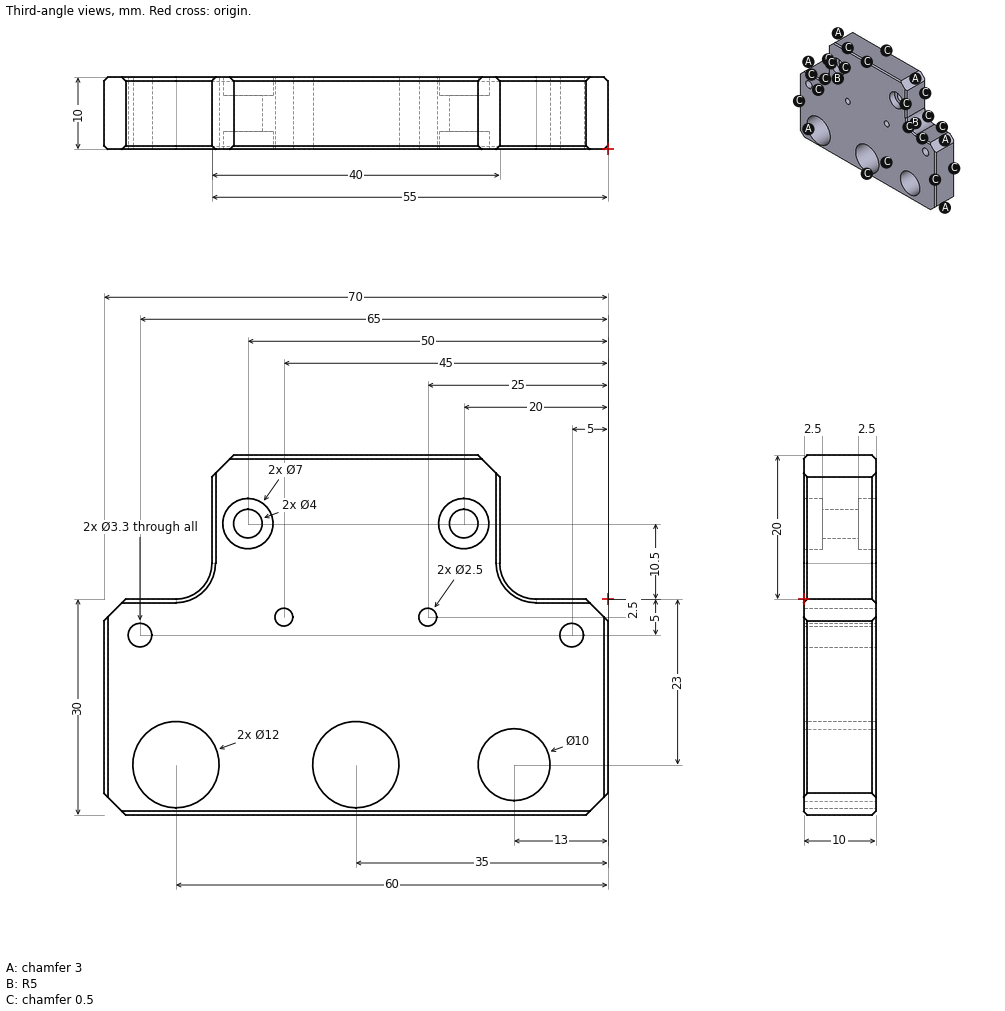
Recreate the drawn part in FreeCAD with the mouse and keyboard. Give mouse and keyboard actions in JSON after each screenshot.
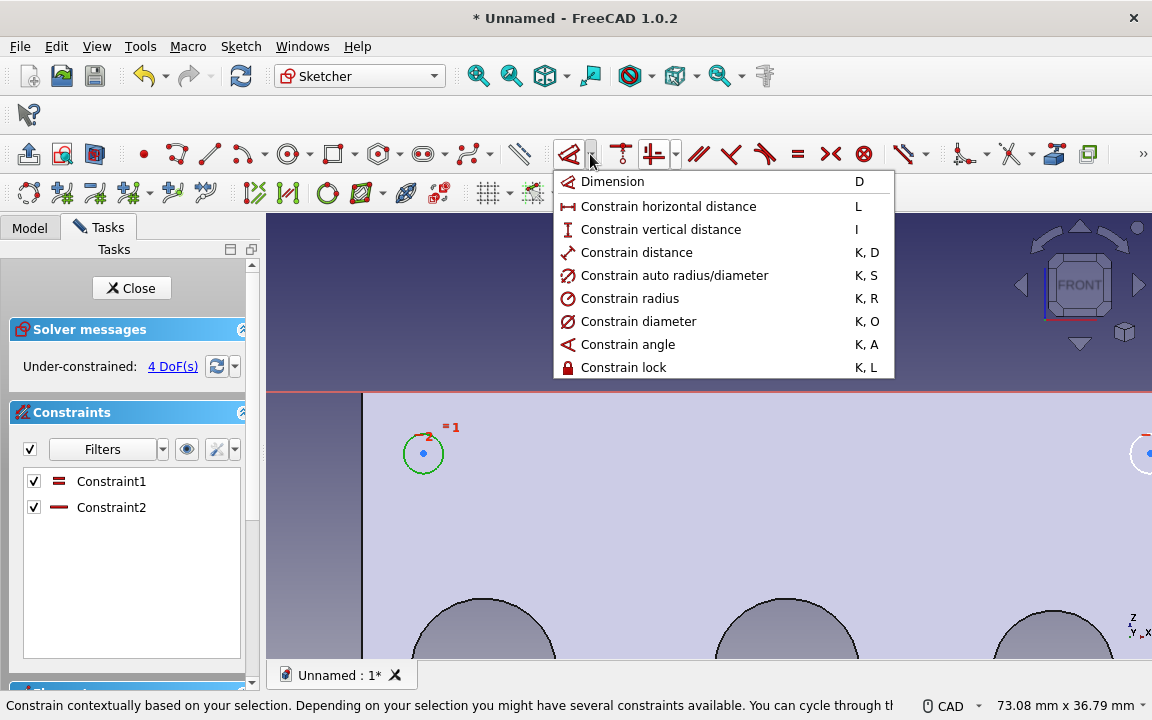
{"action": "left_click", "coordinate": [724, 322]}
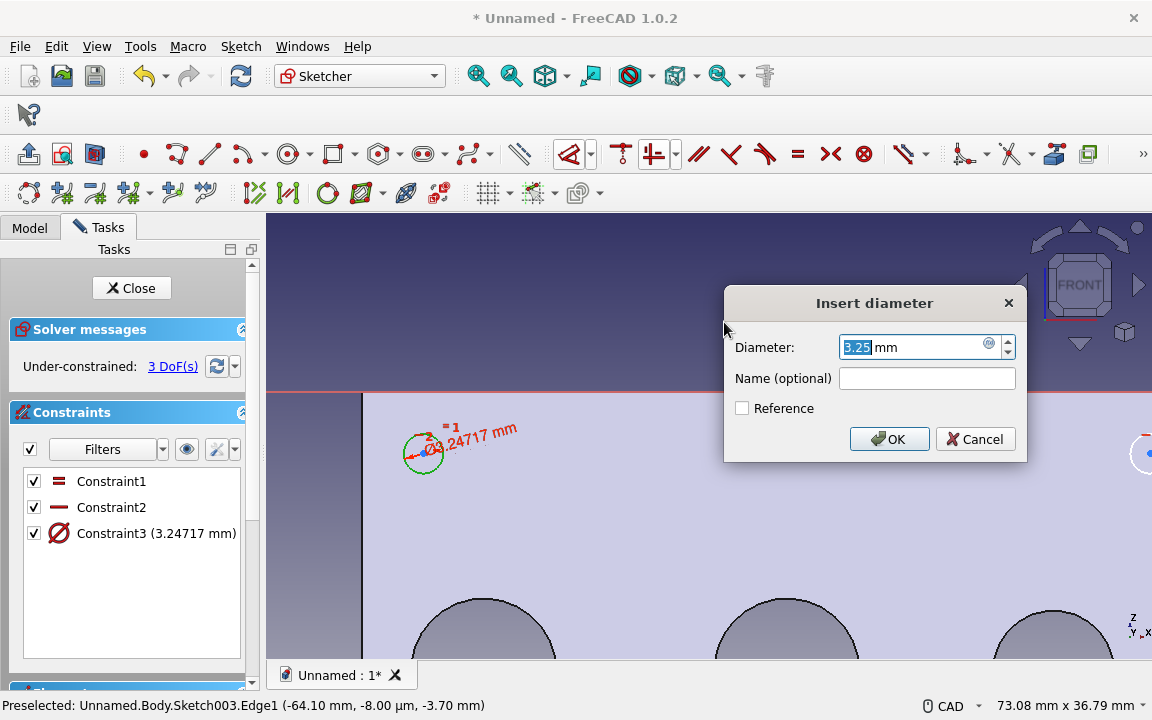
{"action": "type", "text": "3.3"}
{"action": "key", "text": "Return"}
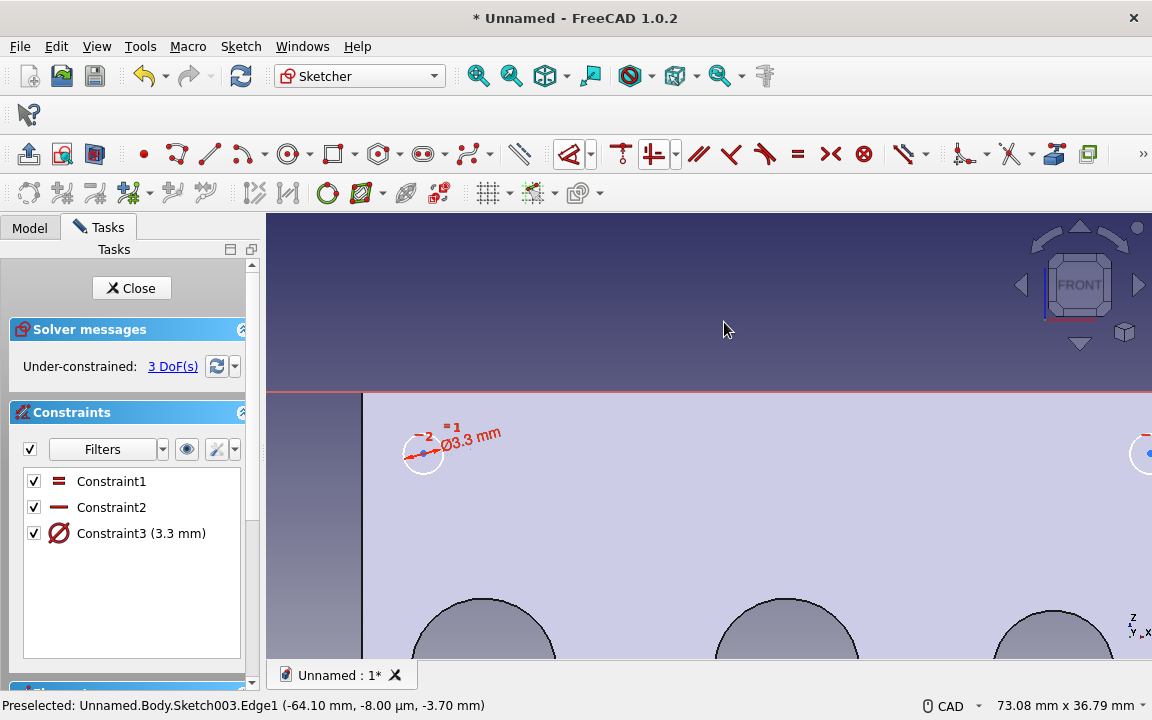
{"action": "left_click", "coordinate": [423, 454]}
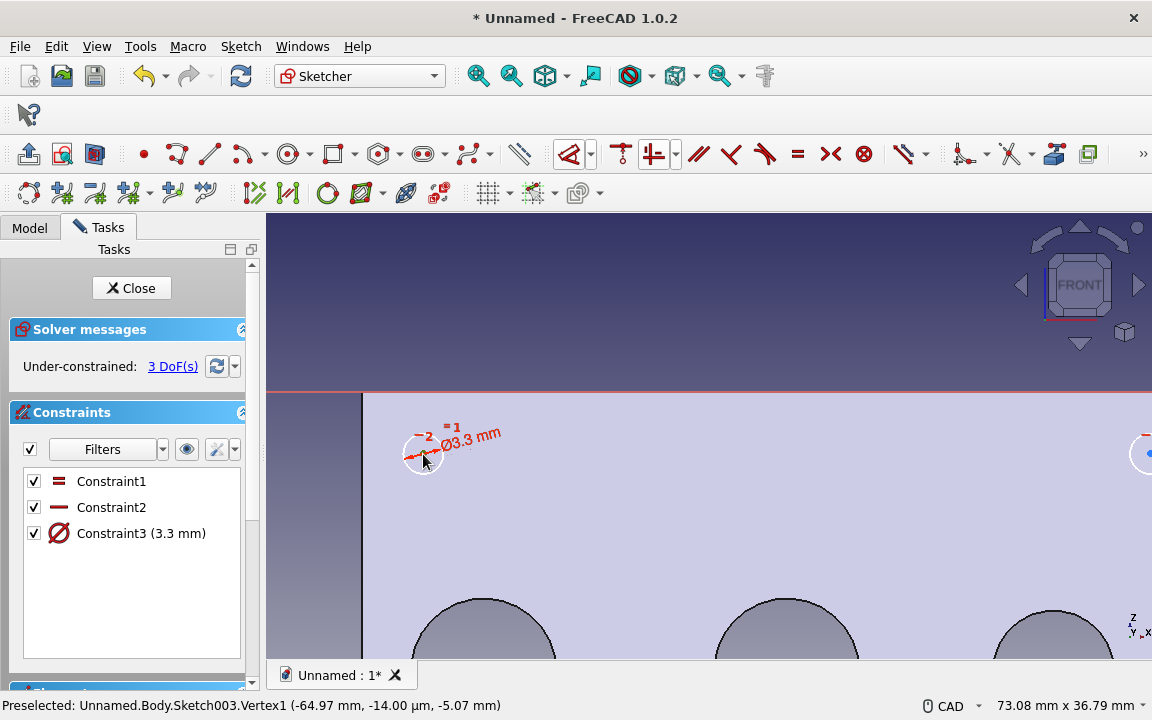
{"action": "left_click", "coordinate": [590, 154]}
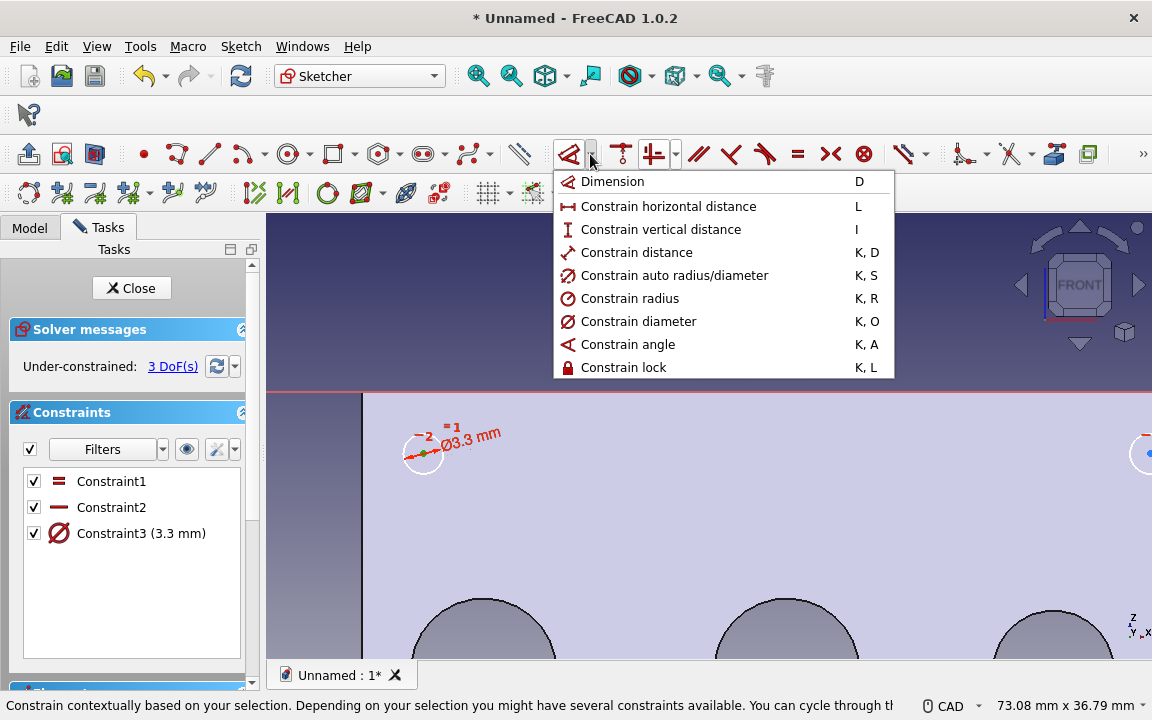
{"action": "left_click", "coordinate": [724, 230]}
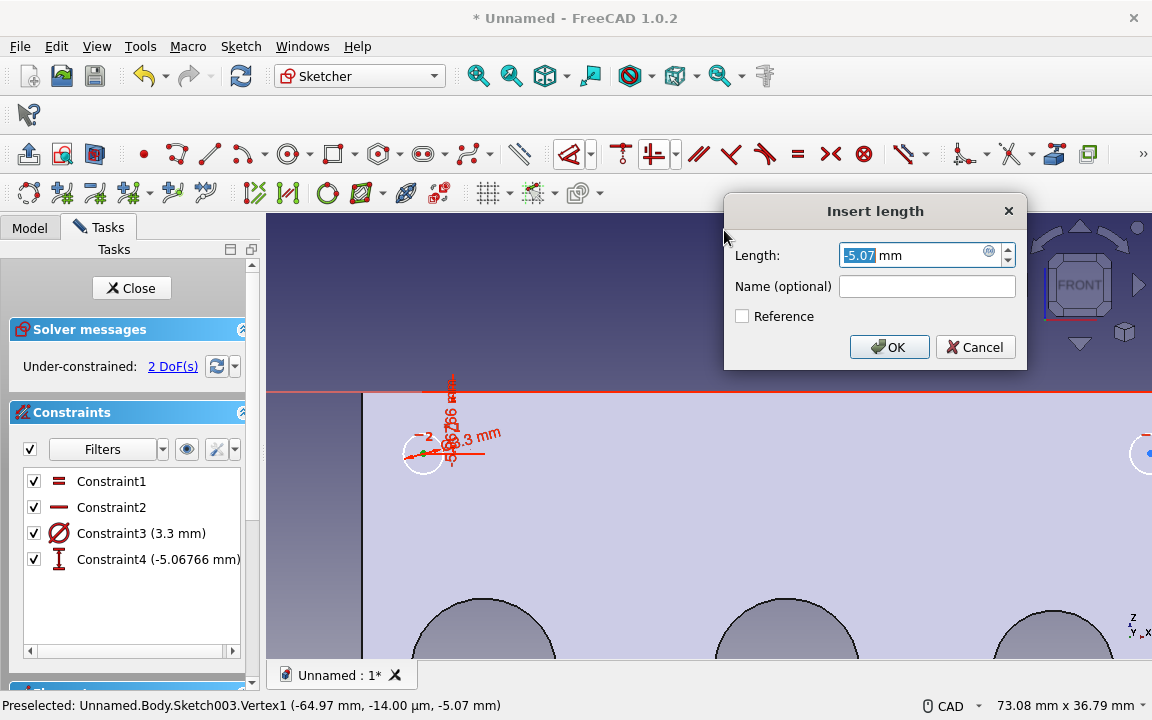
{"action": "type", "text": "-5"}
{"action": "key", "text": "Return"}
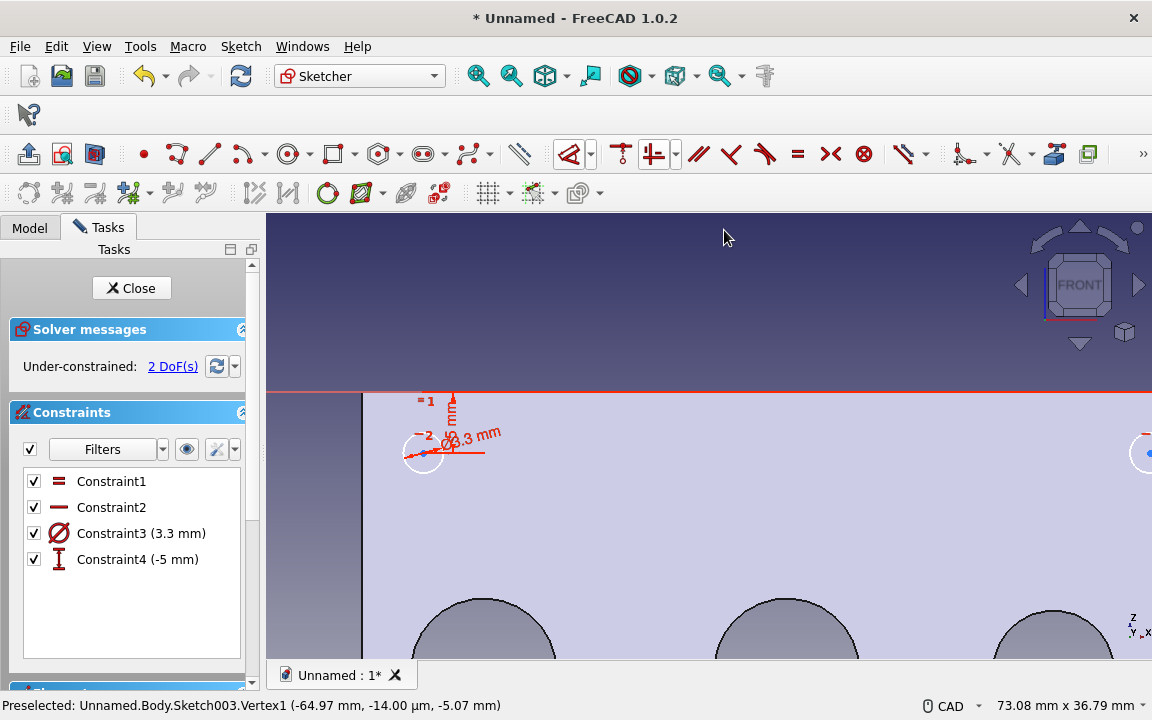
{"action": "scroll", "coordinate": [438, 440], "scroll_direction": "down", "scroll_amount": 3}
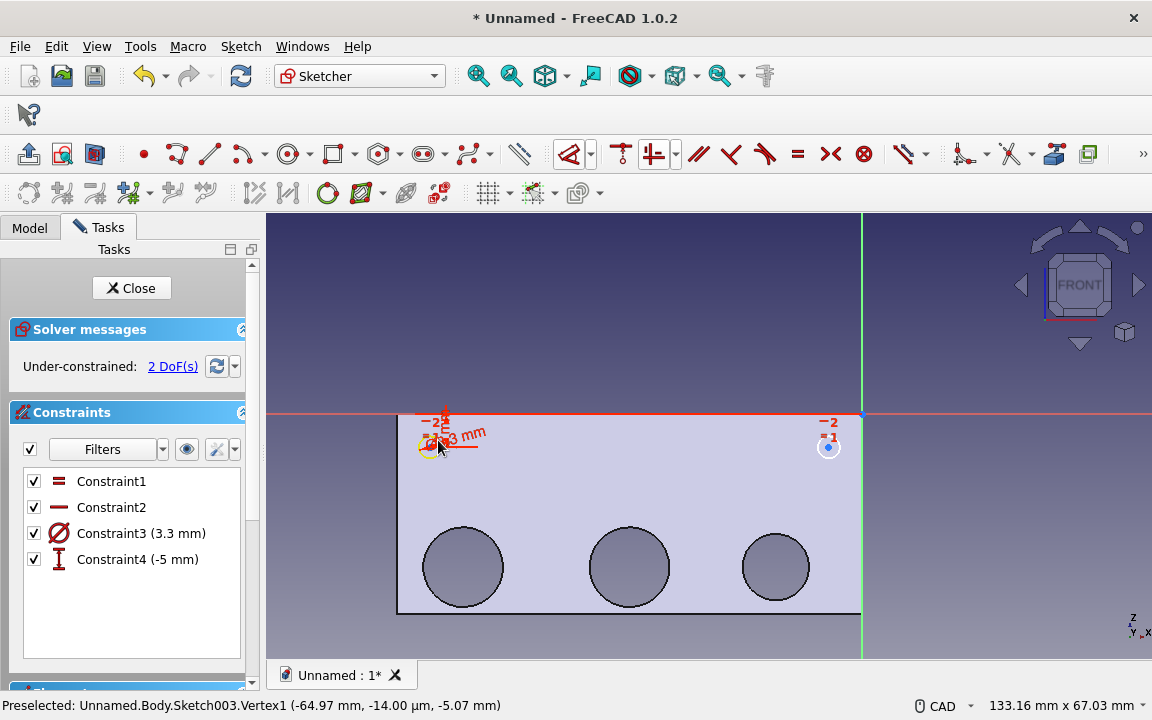
{"action": "left_click", "coordinate": [829, 447]}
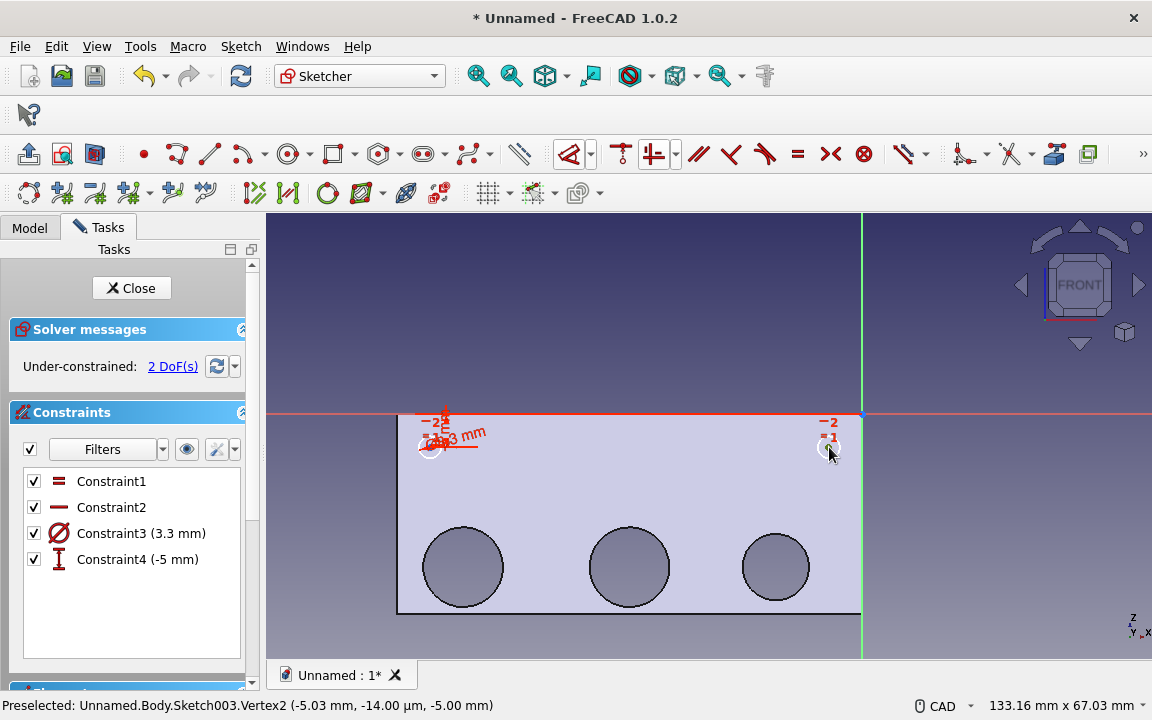
{"action": "left_click", "coordinate": [590, 154]}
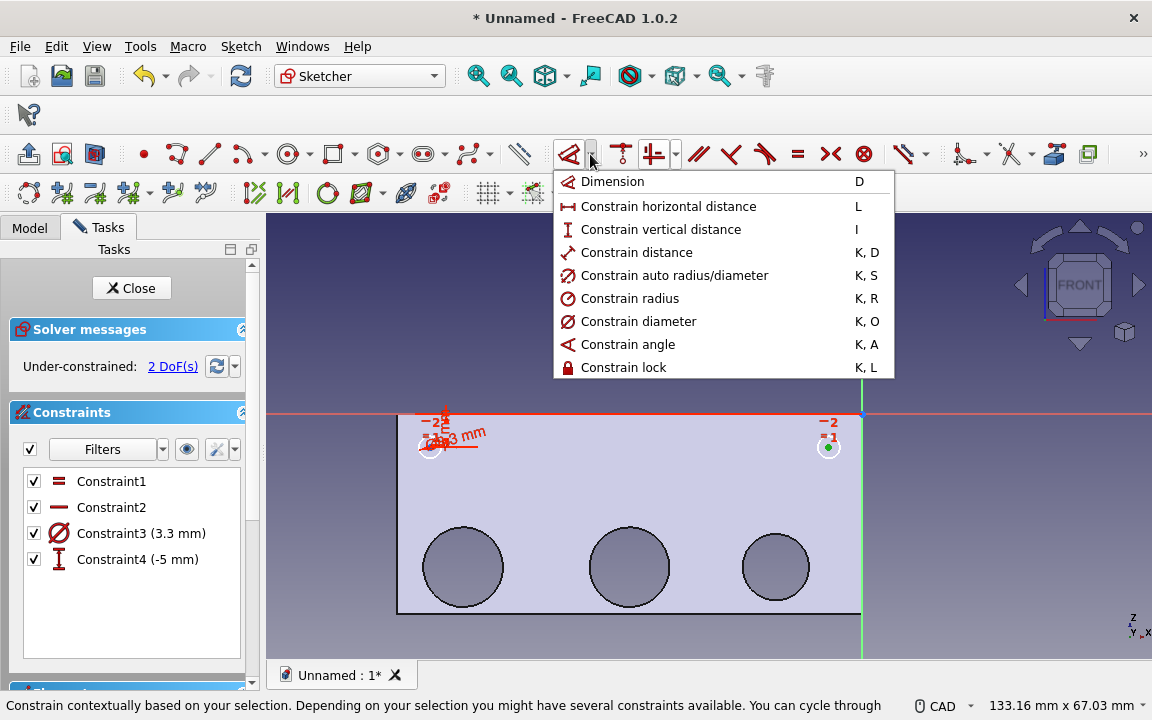
{"action": "left_click", "coordinate": [724, 206]}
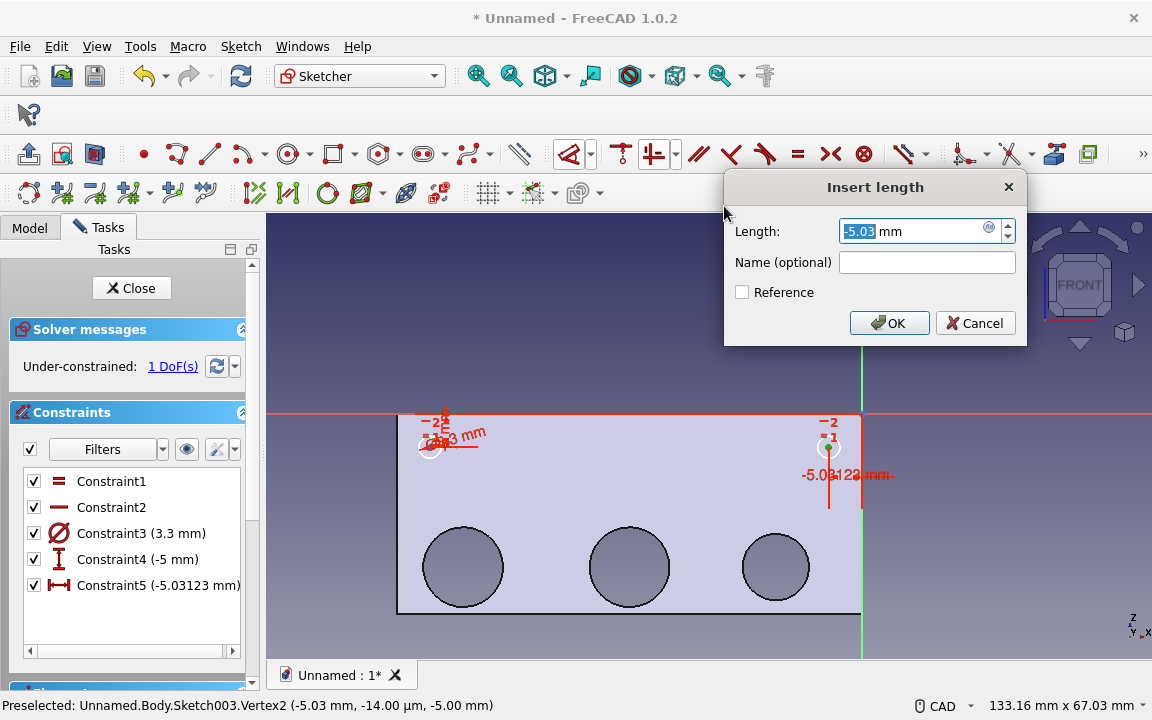
{"action": "type", "text": "-5"}
{"action": "key", "text": "Return"}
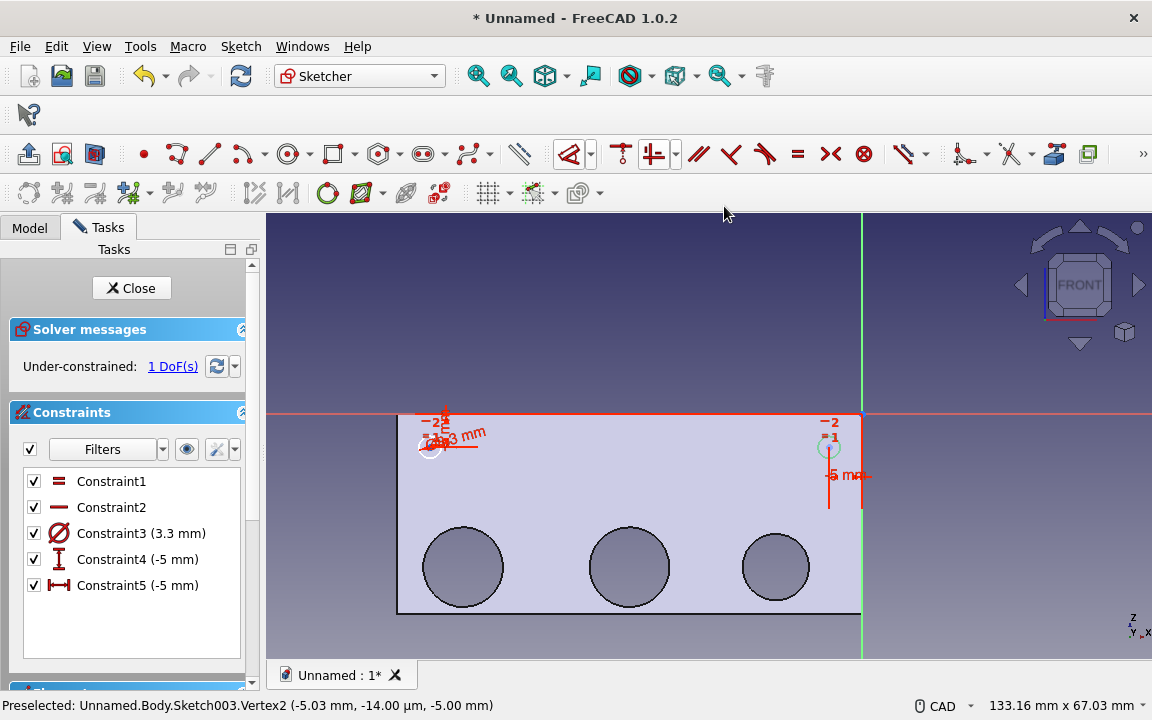
{"action": "left_click", "coordinate": [430, 447]}